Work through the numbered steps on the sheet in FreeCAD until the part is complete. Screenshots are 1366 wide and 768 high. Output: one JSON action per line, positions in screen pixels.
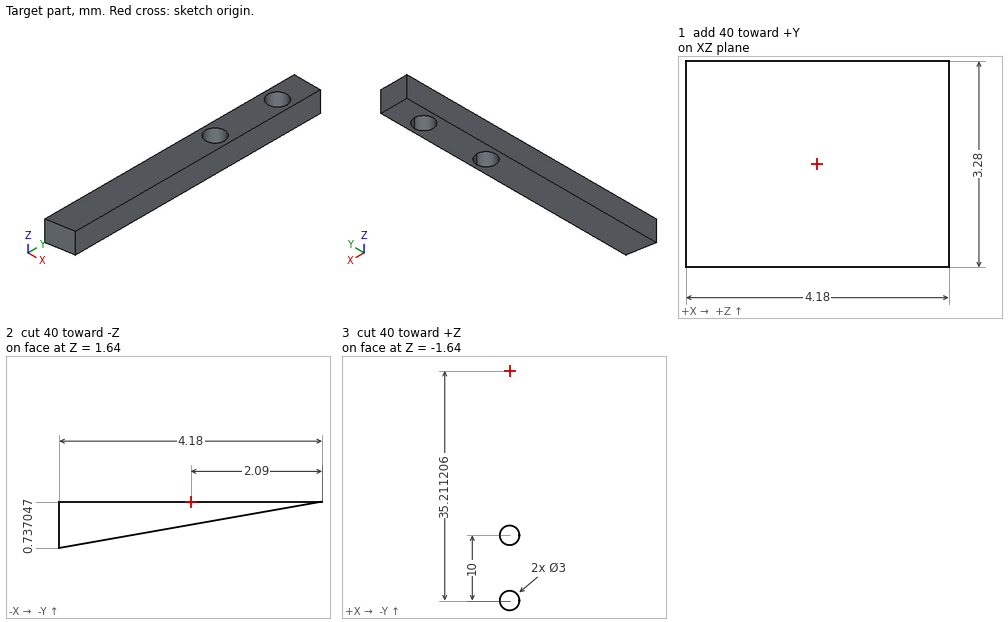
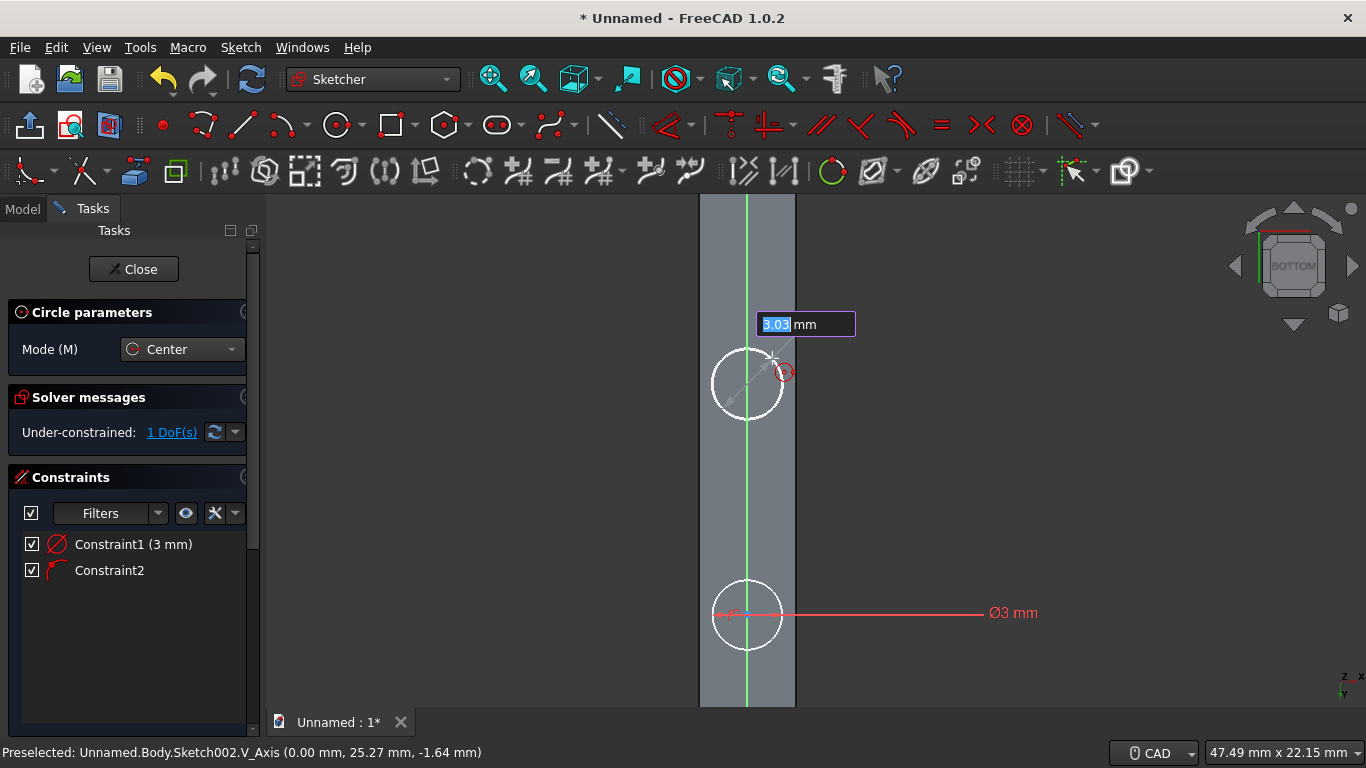
{"action": "type", "text": "3"}
{"action": "key", "text": "Return"}
{"action": "key", "text": "Escape"}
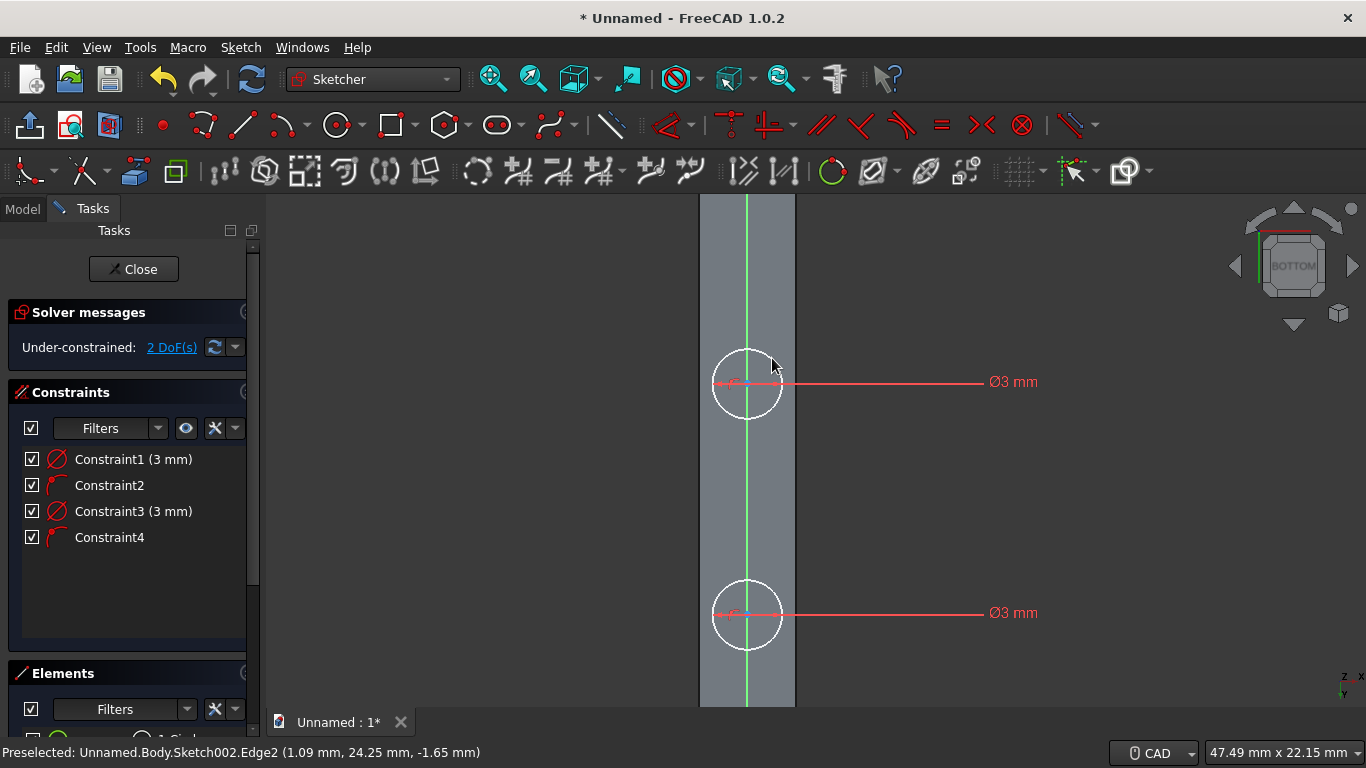
{"action": "left_click", "coordinate": [666, 126]}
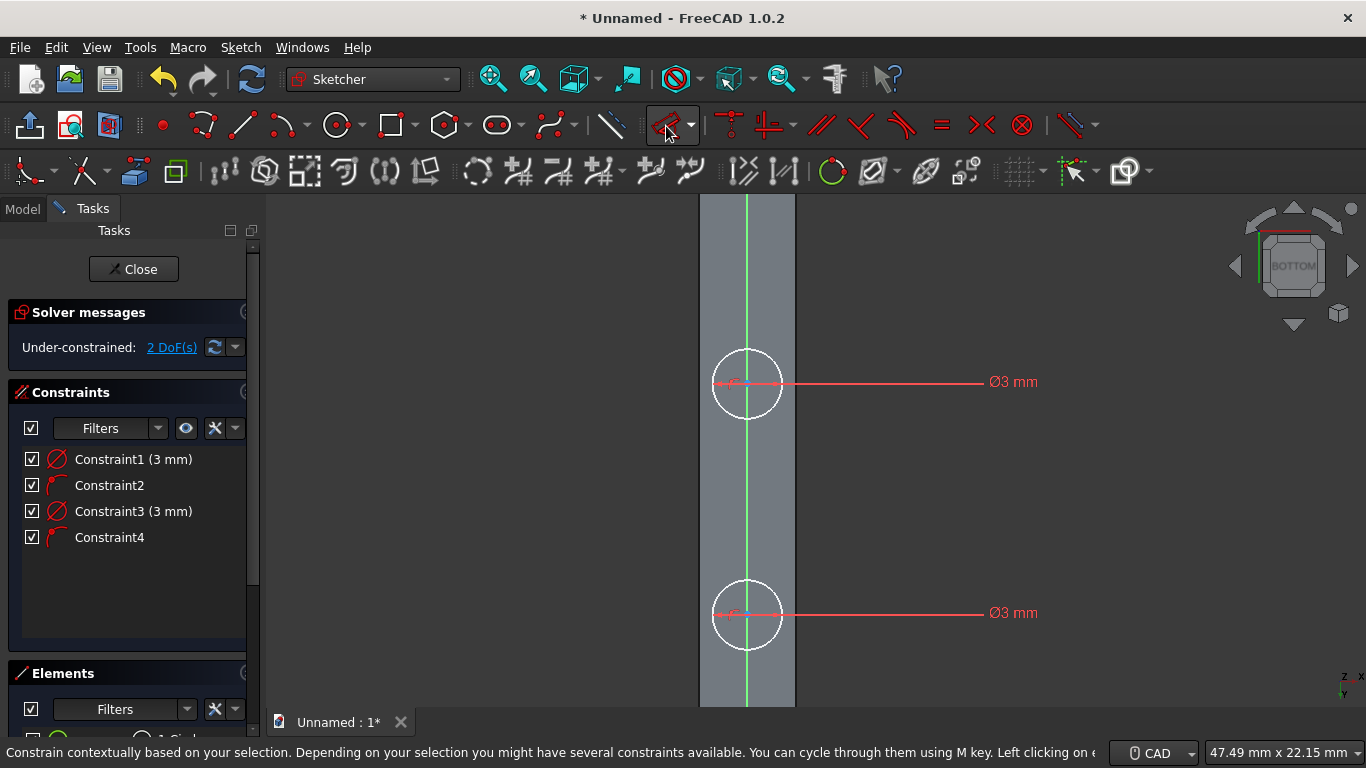
{"action": "left_click", "coordinate": [747, 615]}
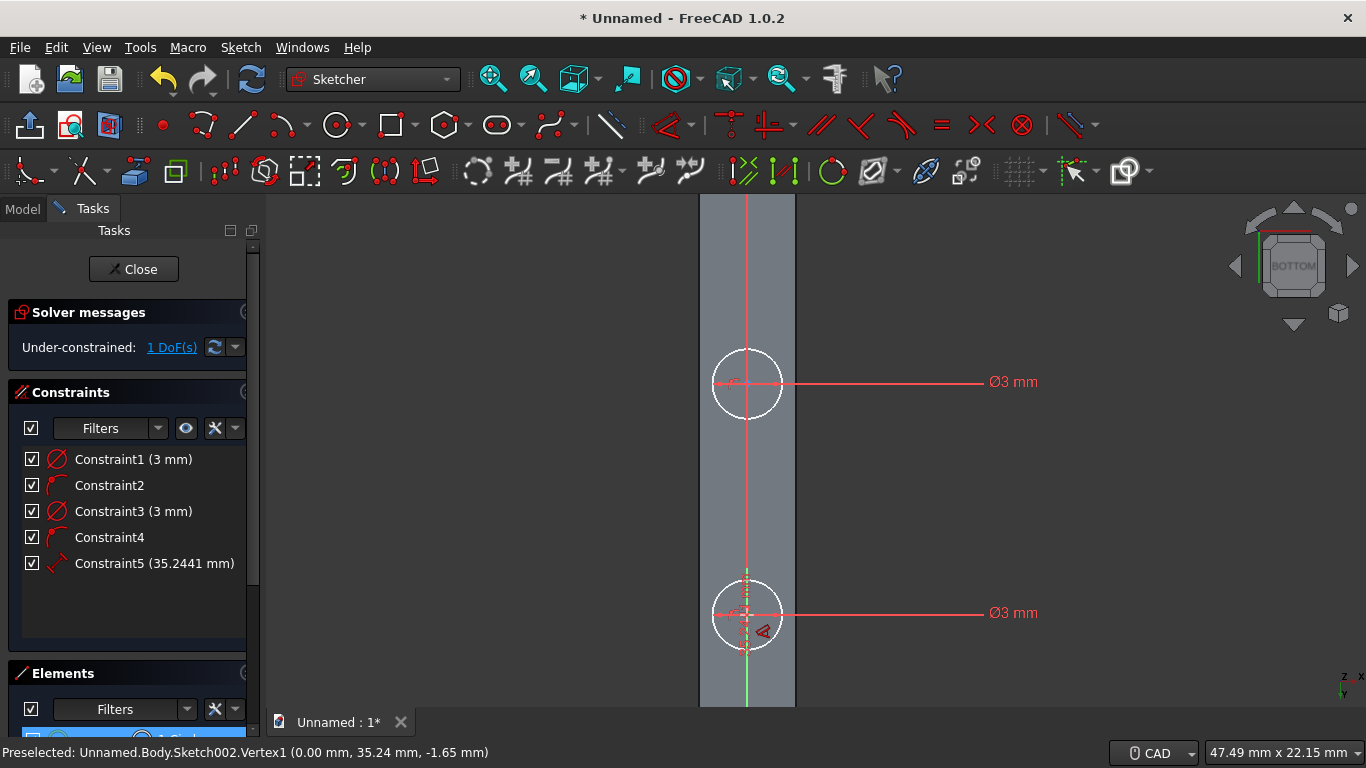
{"action": "left_click", "coordinate": [747, 384]}
{"action": "left_click", "coordinate": [781, 500]}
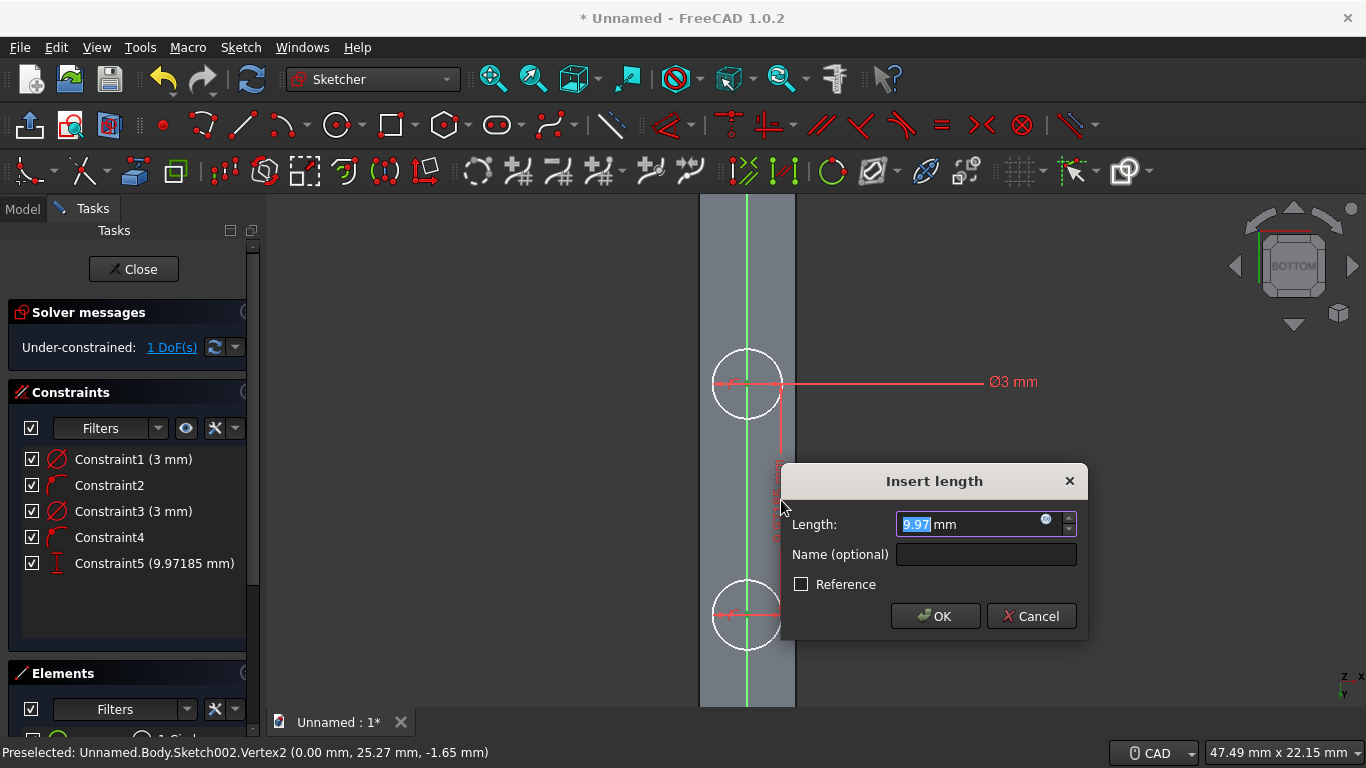
{"action": "type", "text": "10"}
{"action": "key", "text": "Return"}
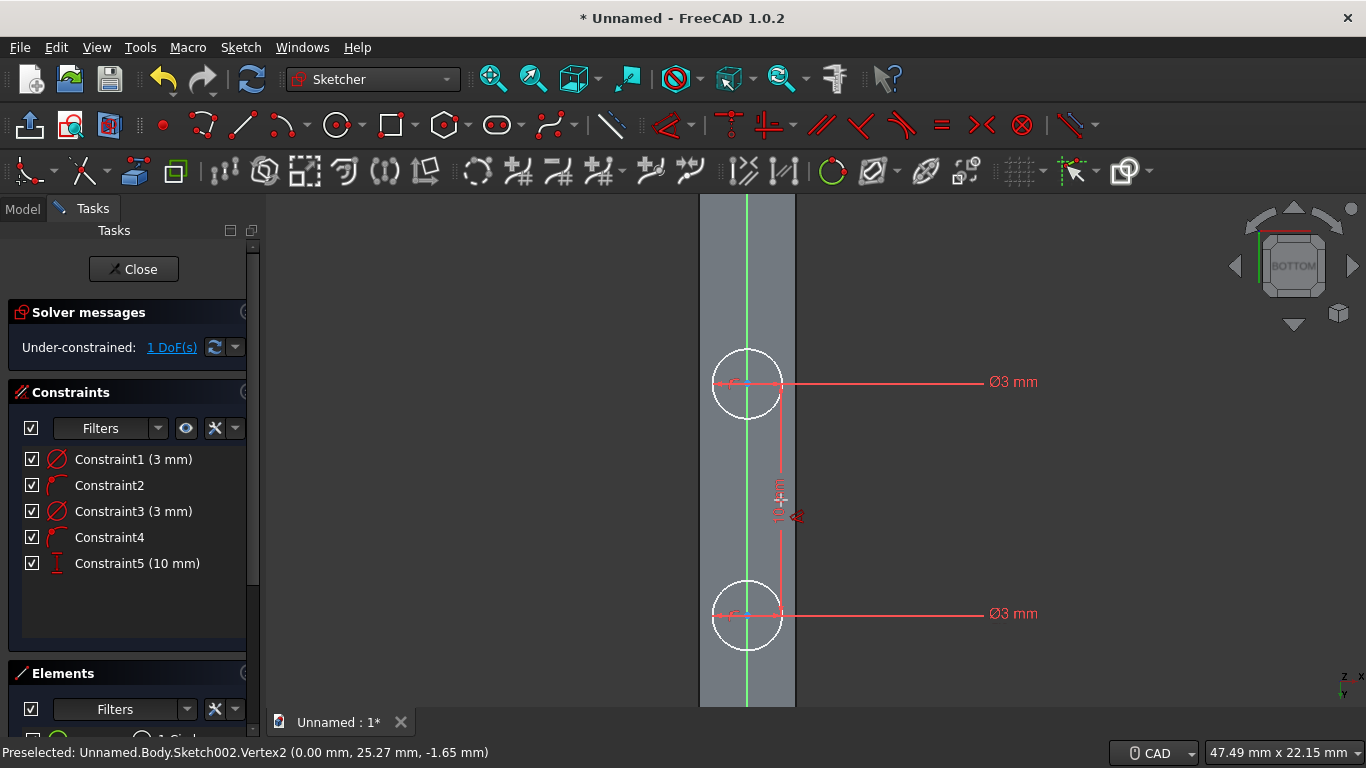
{"action": "left_click", "coordinate": [747, 616]}
{"action": "left_click", "coordinate": [781, 419]}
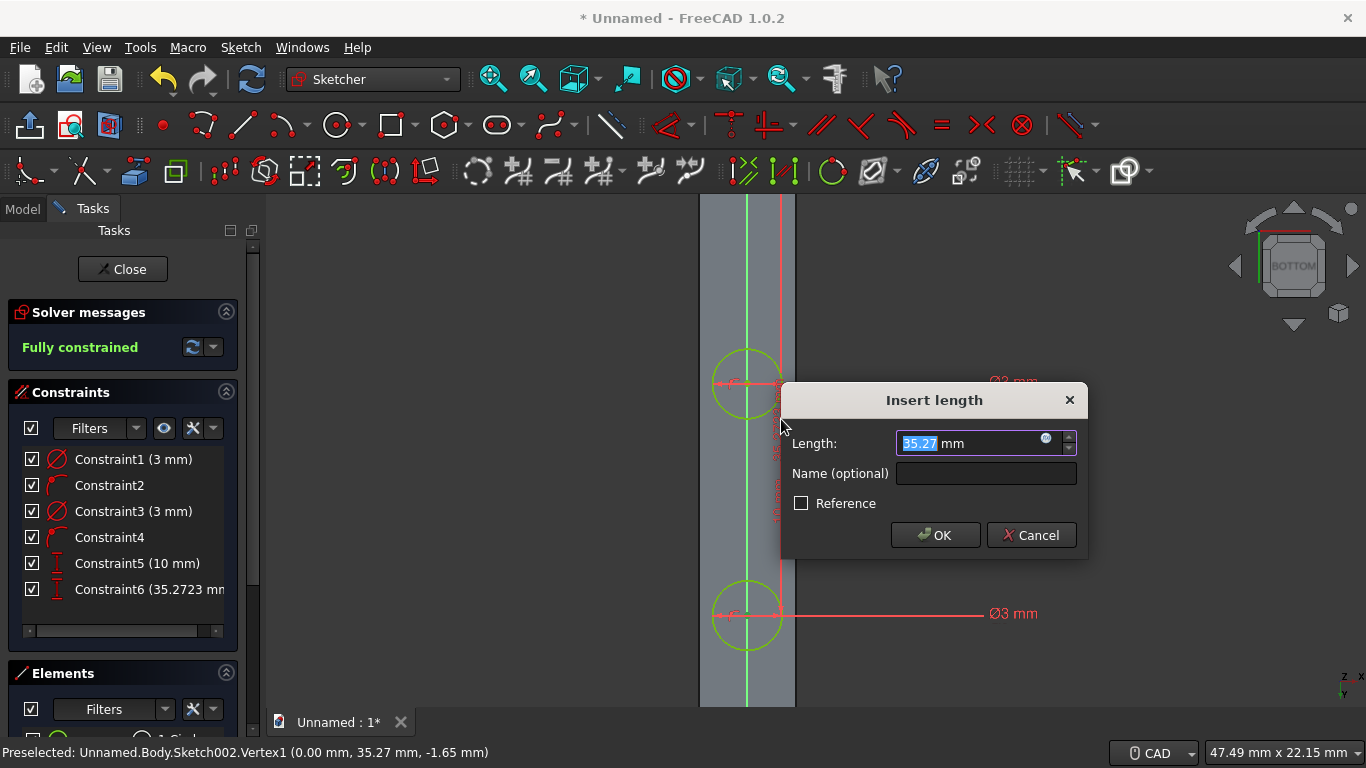
{"action": "type", "text": "35.211206"}
{"action": "key", "text": "Return"}
{"action": "key", "text": "Escape"}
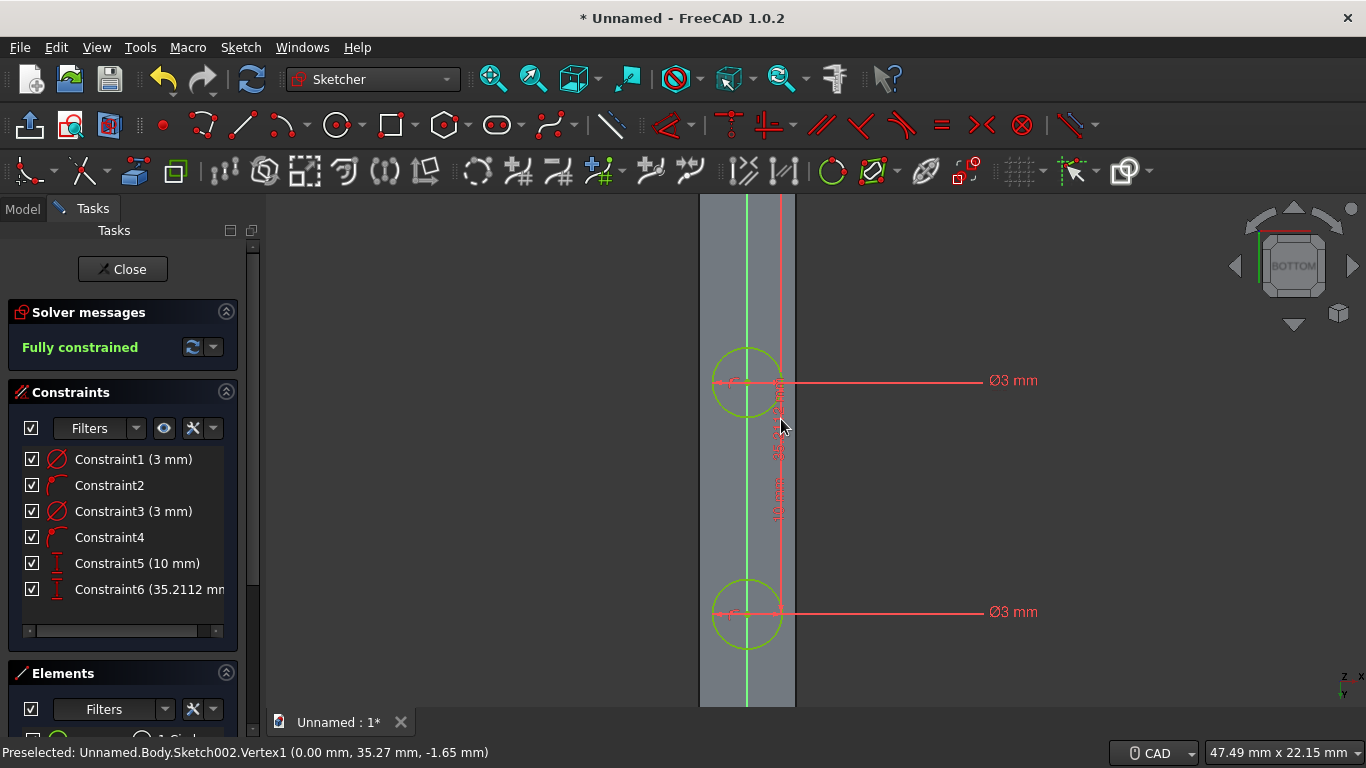
{"action": "left_click", "coordinate": [123, 269]}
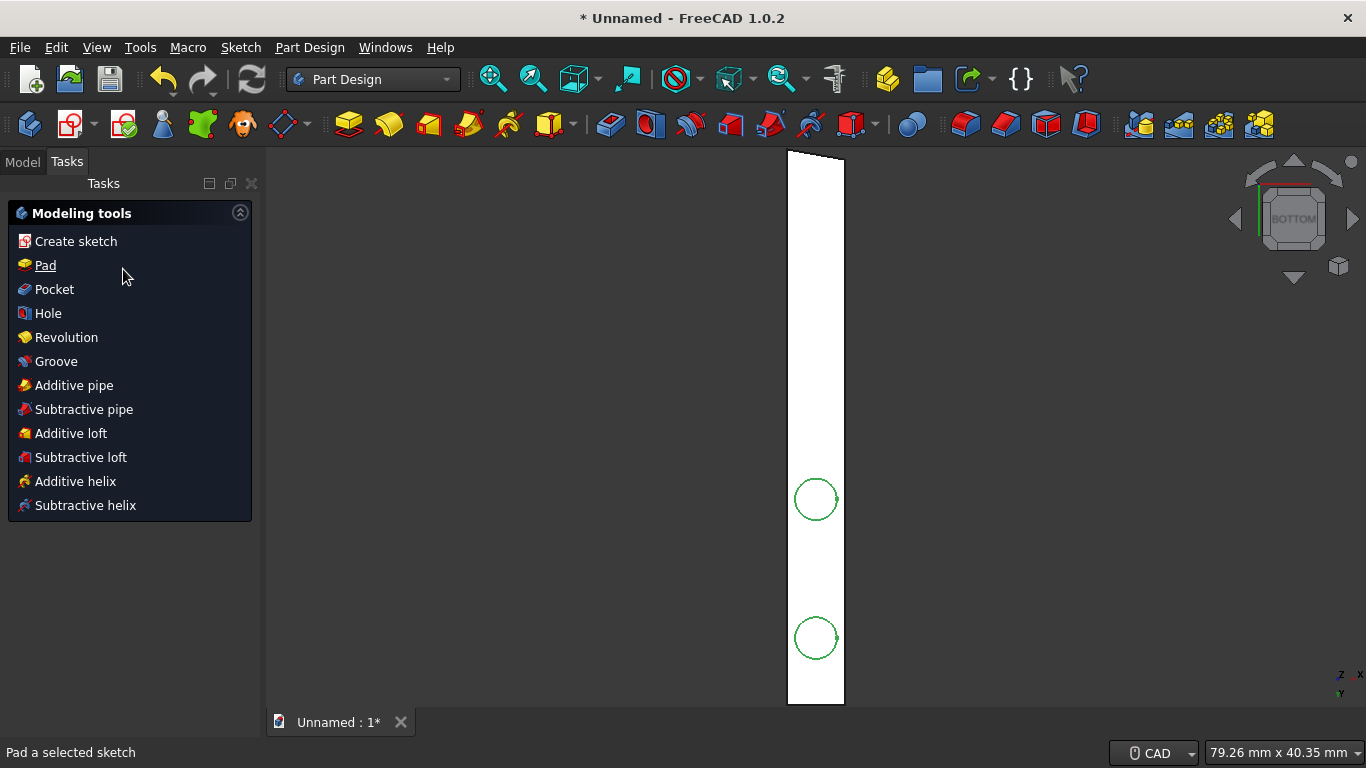
{"action": "left_click", "coordinate": [612, 124]}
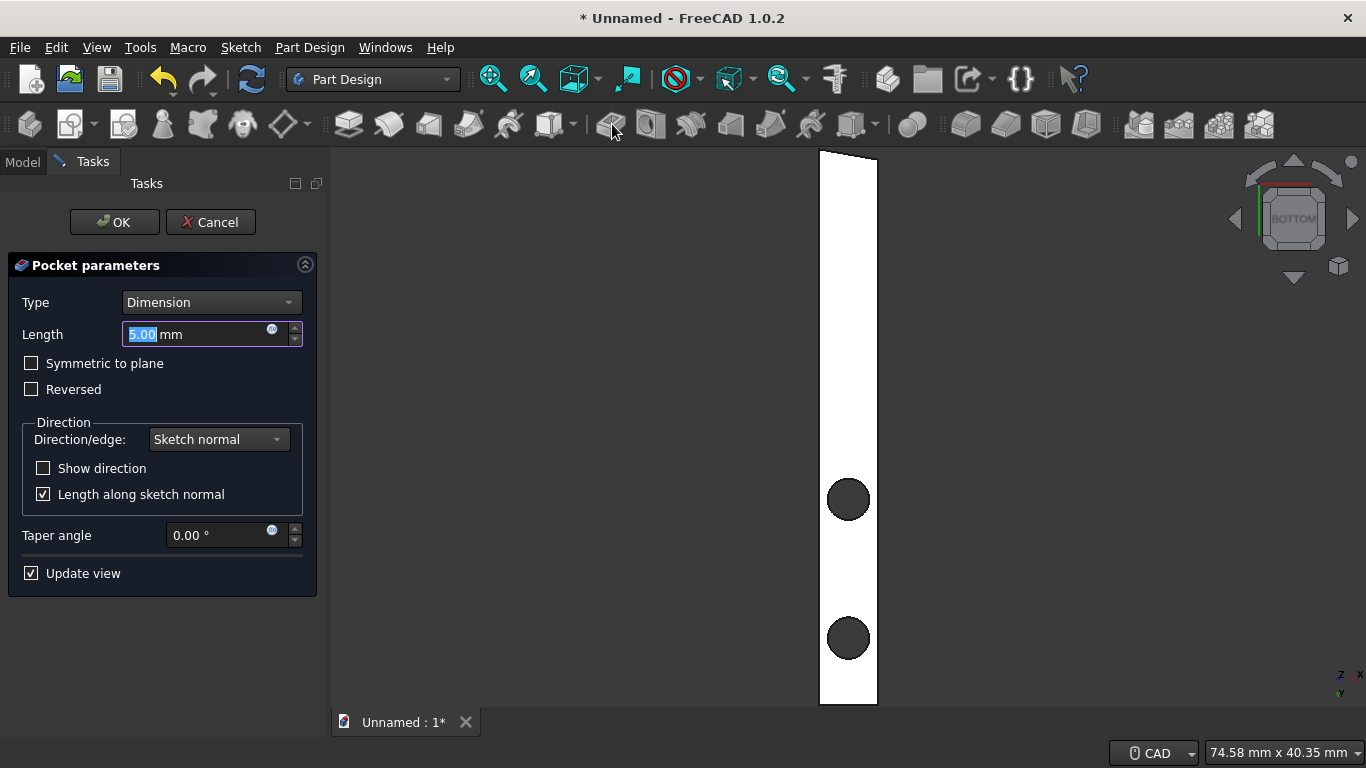
{"action": "type", "text": "40"}
{"action": "key", "text": "Tab"}